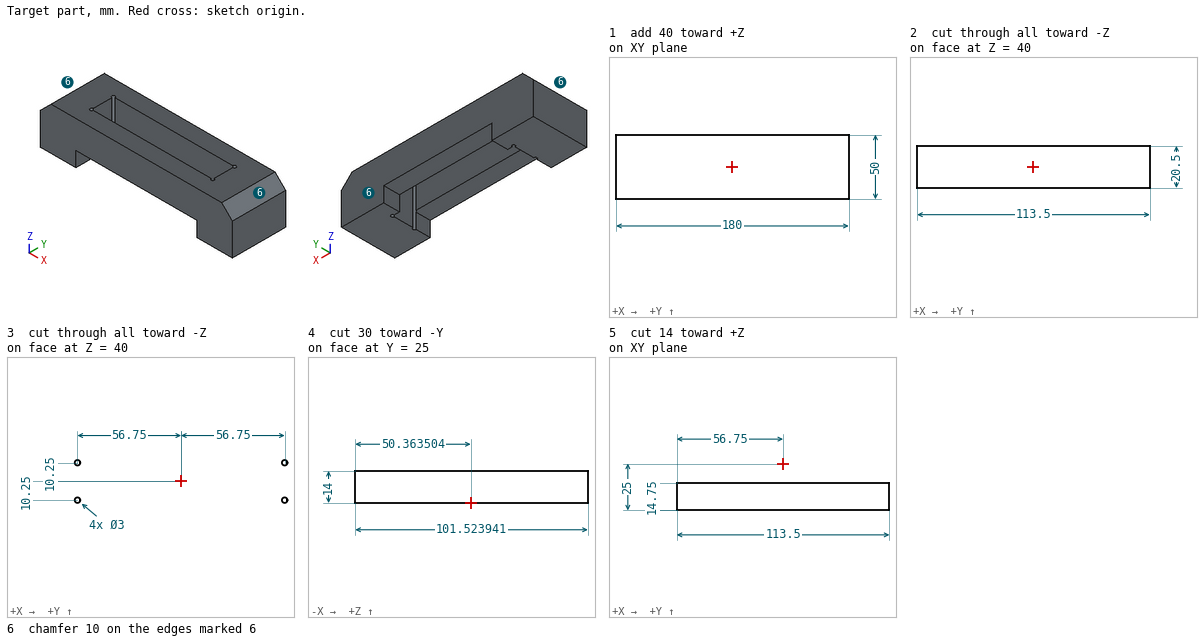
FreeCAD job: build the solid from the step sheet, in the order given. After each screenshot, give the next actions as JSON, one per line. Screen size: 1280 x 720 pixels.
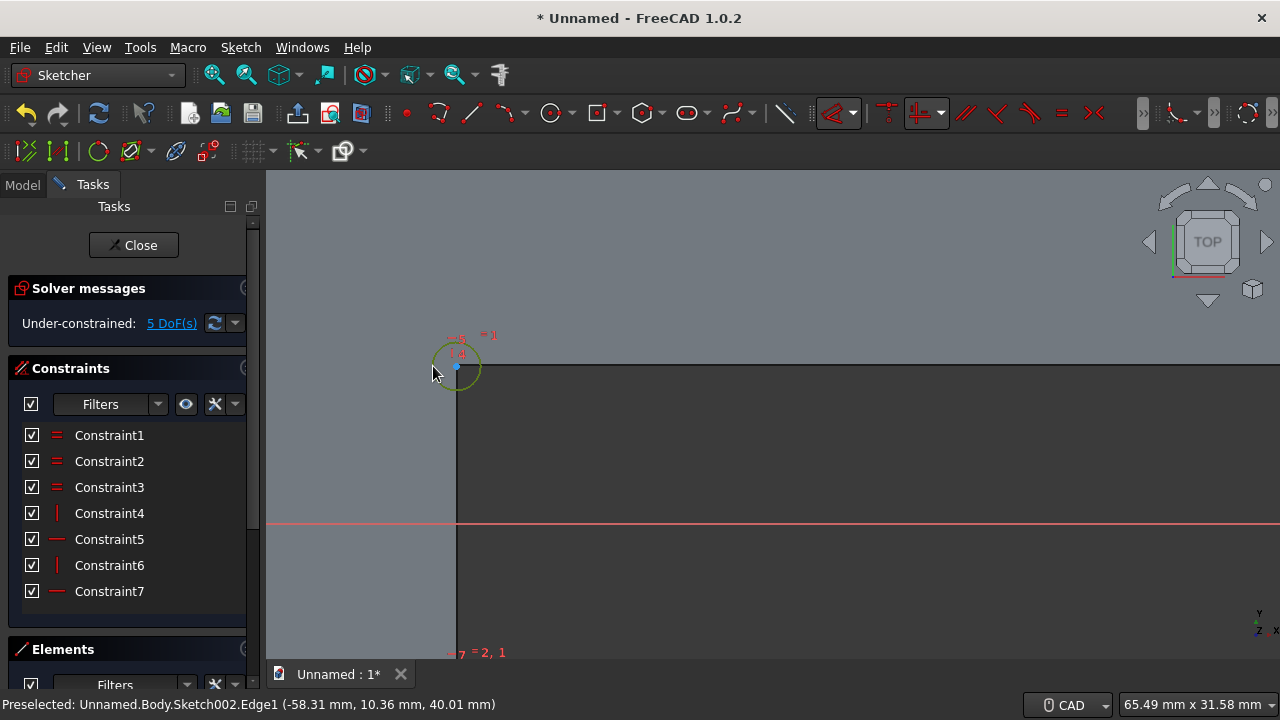
{"action": "left_click", "coordinate": [856, 114]}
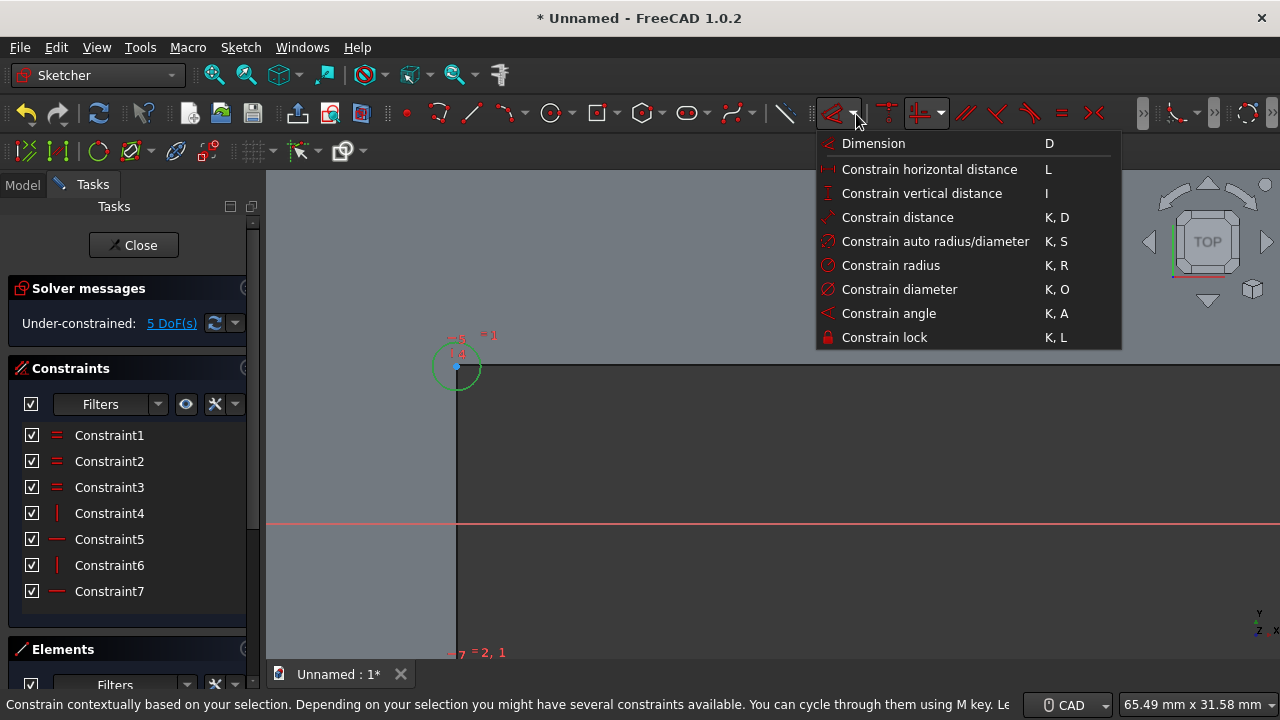
{"action": "left_click", "coordinate": [969, 289]}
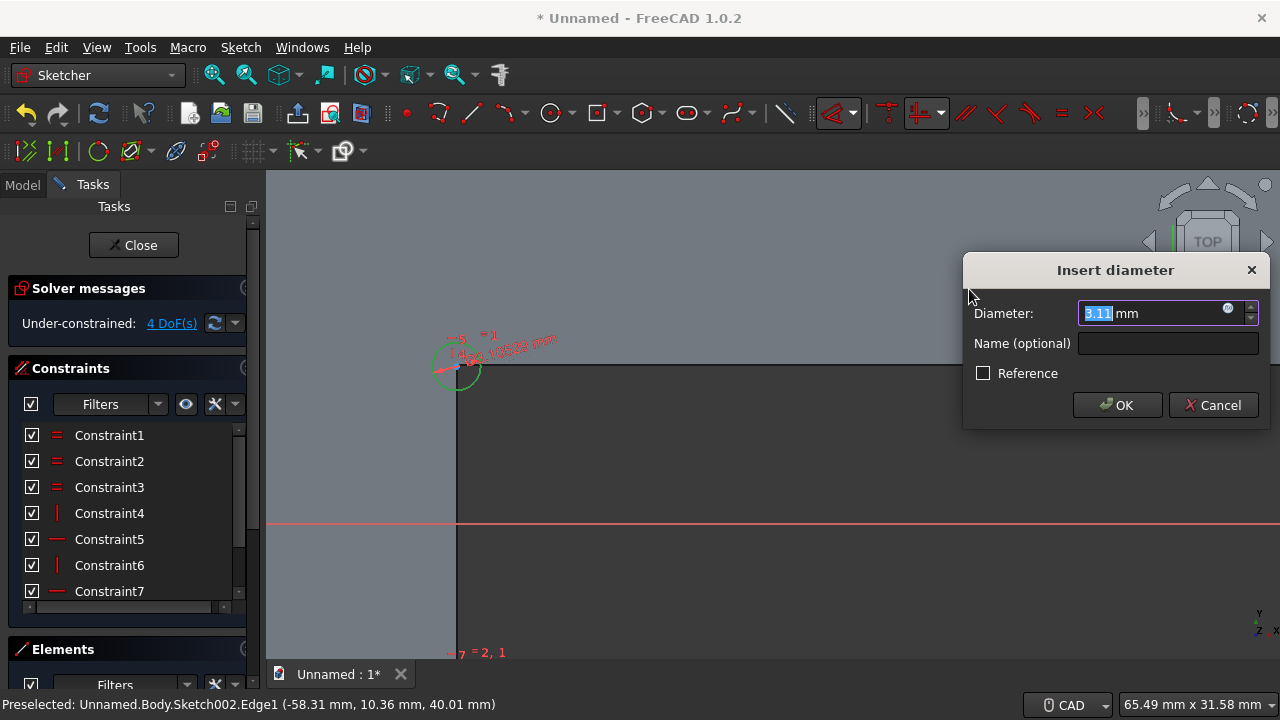
{"action": "type", "text": "3"}
{"action": "key", "text": "Return"}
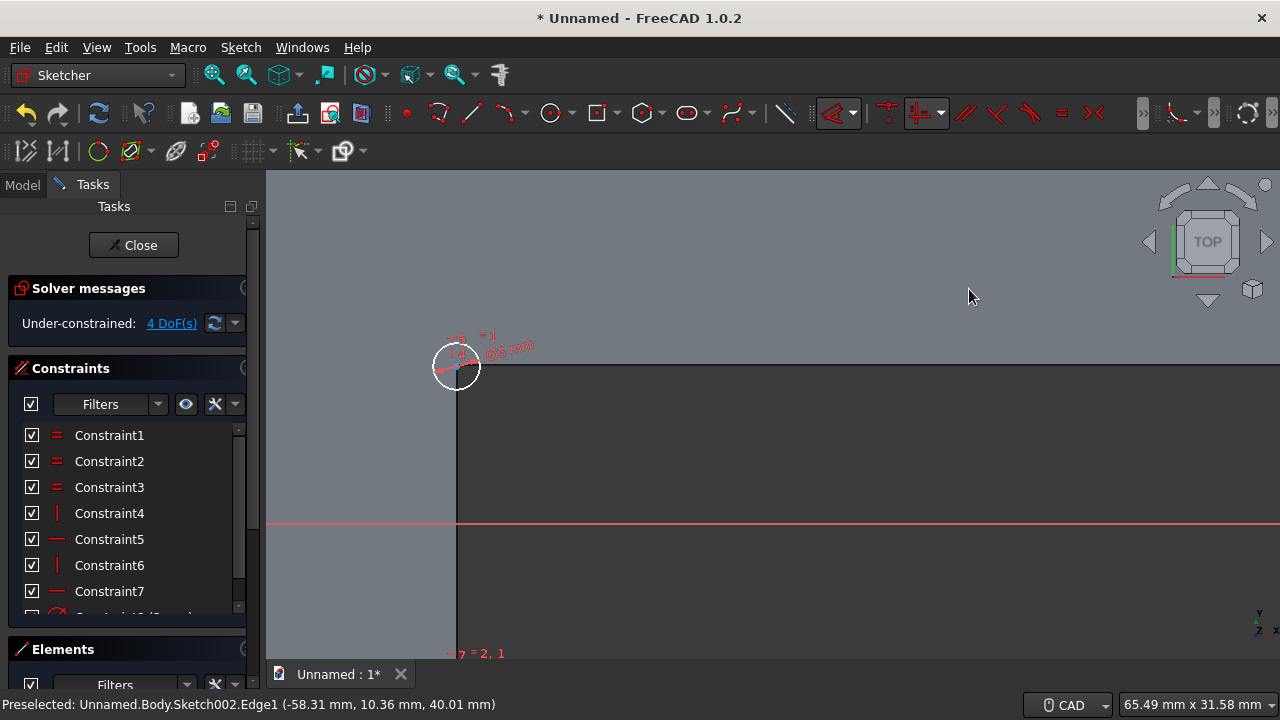
{"action": "left_click", "coordinate": [457, 366]}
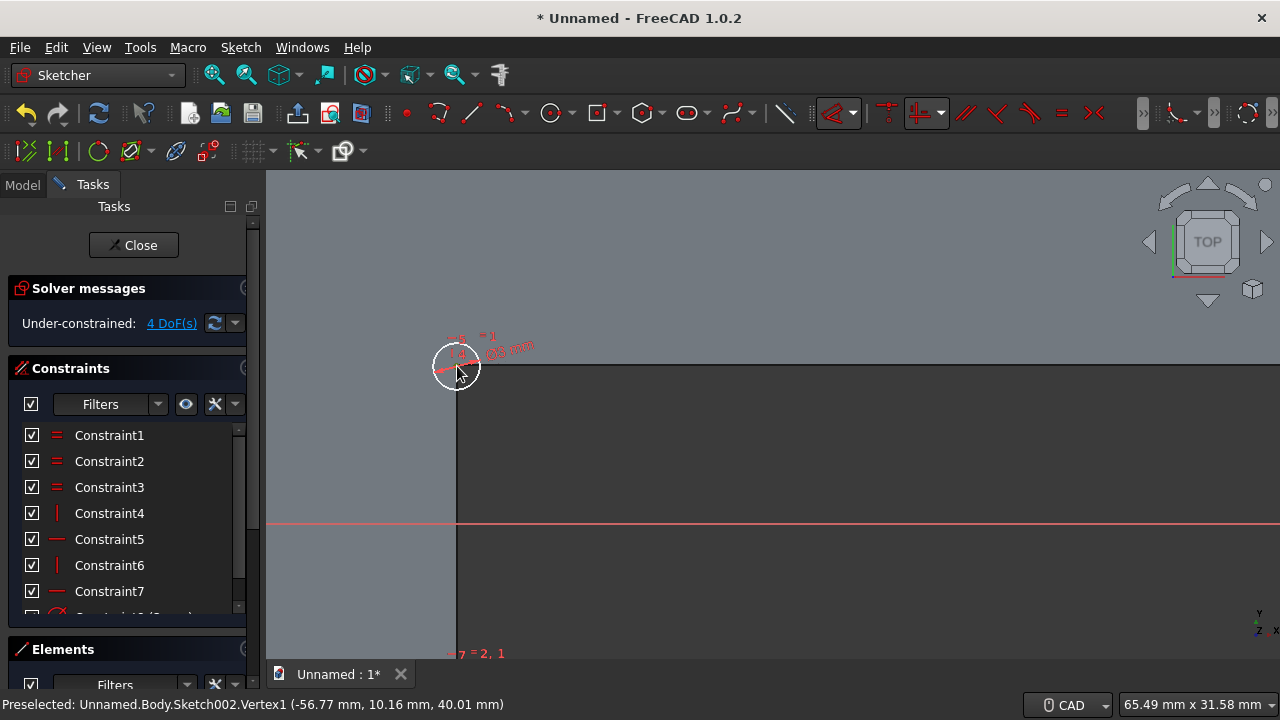
{"action": "left_click", "coordinate": [856, 114]}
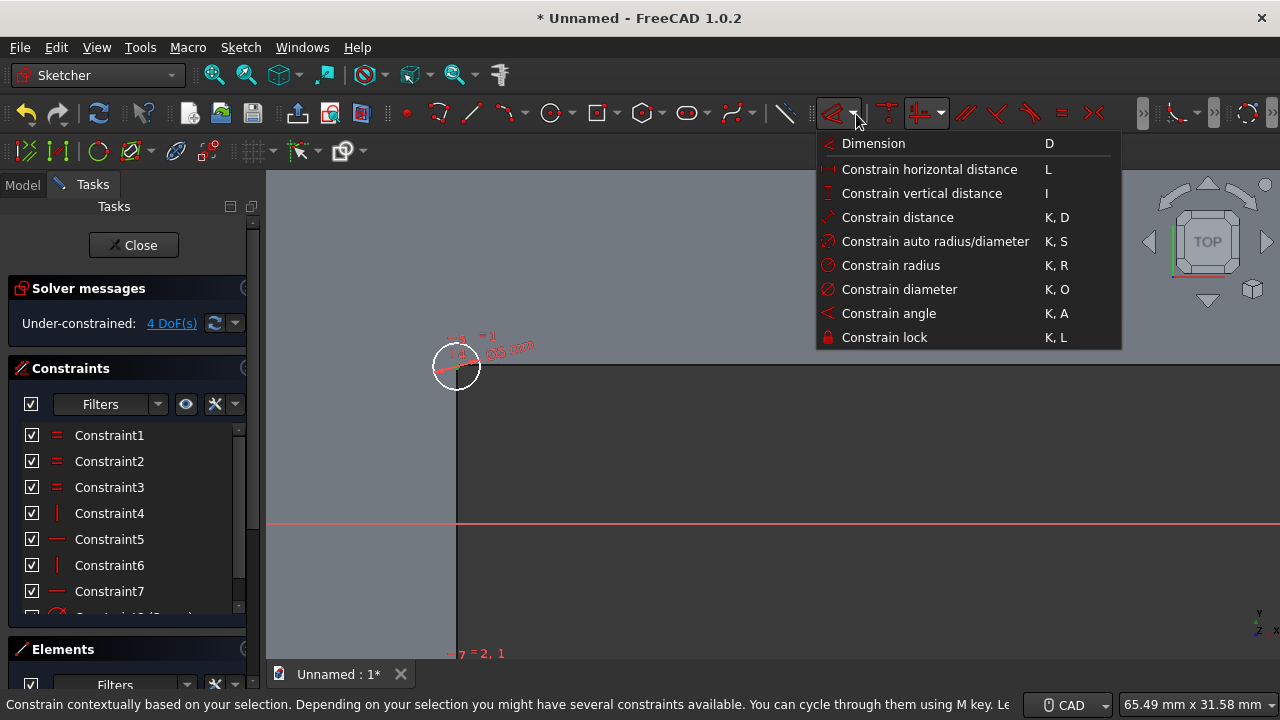
{"action": "left_click", "coordinate": [969, 169]}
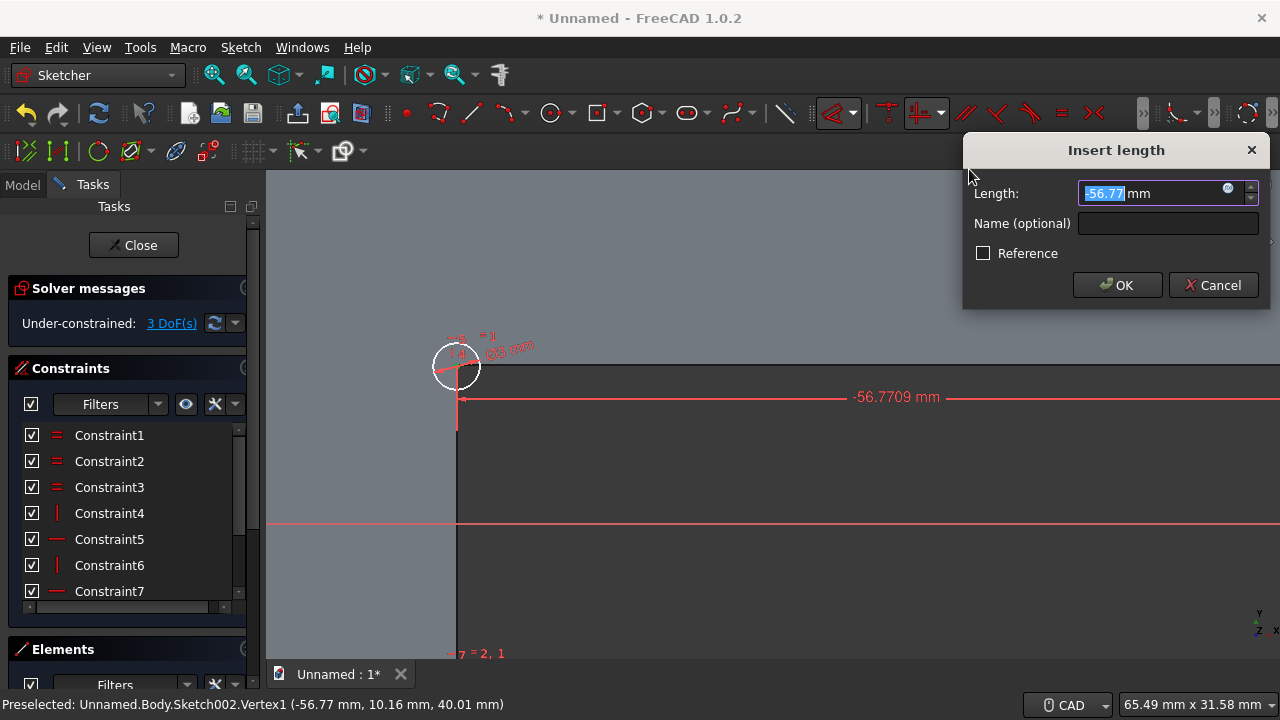
{"action": "type", "text": "-56.75"}
{"action": "key", "text": "Return"}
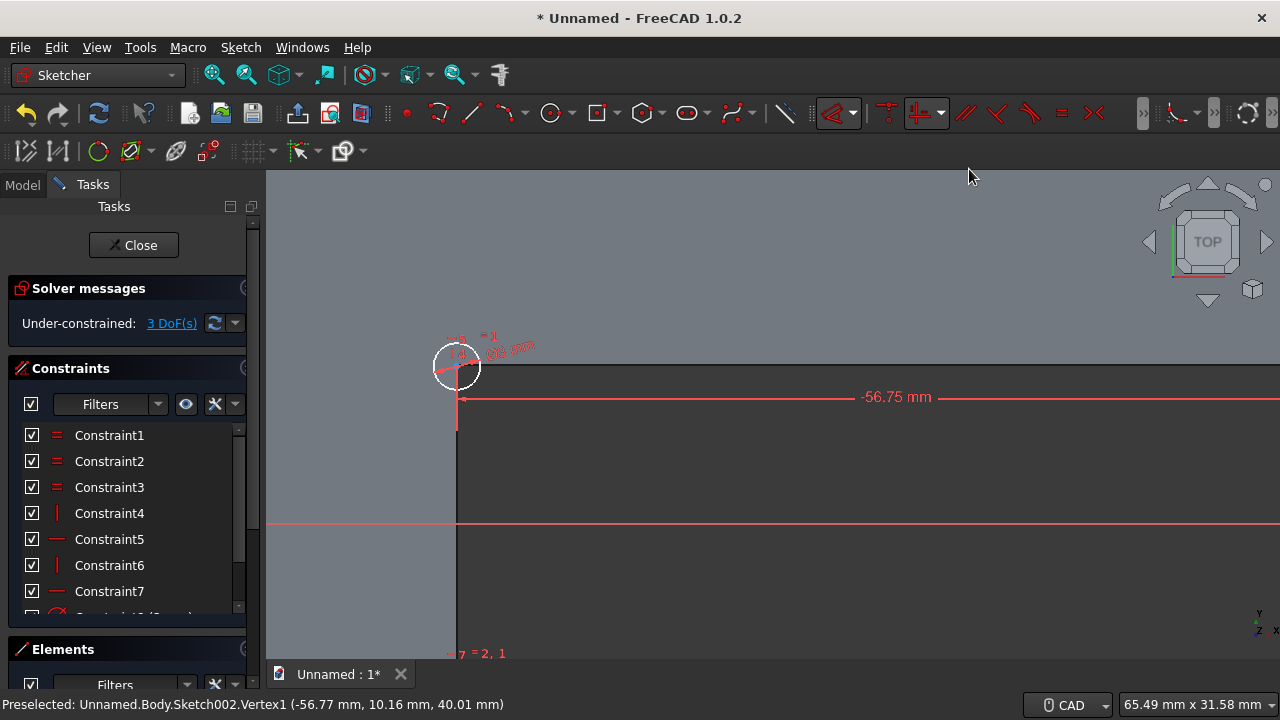
{"action": "left_click", "coordinate": [457, 366]}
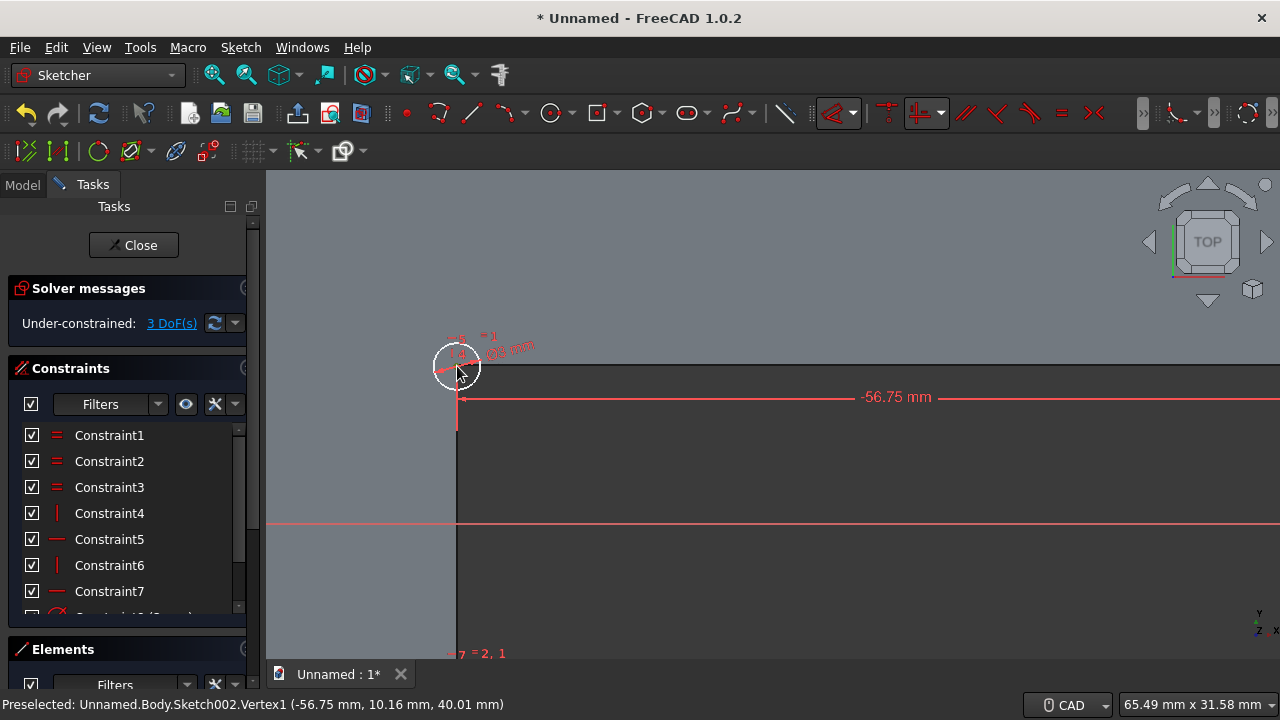
{"action": "left_click", "coordinate": [856, 114]}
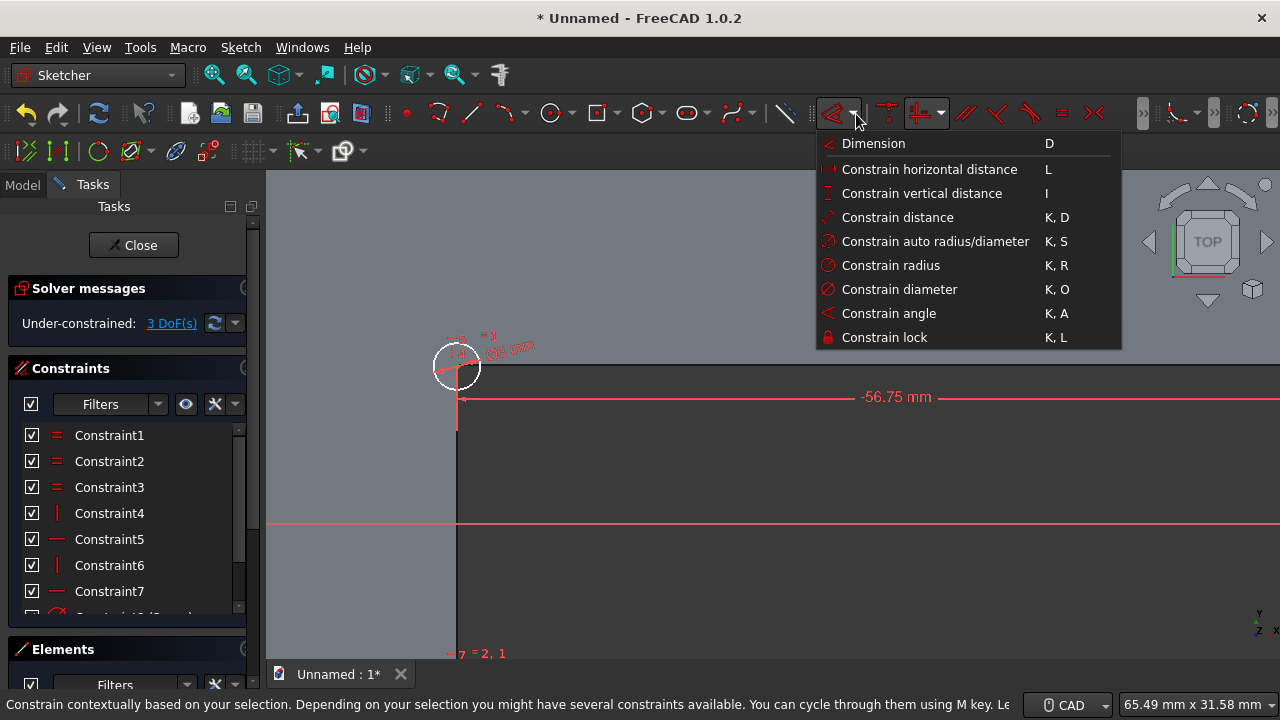
{"action": "left_click", "coordinate": [969, 193]}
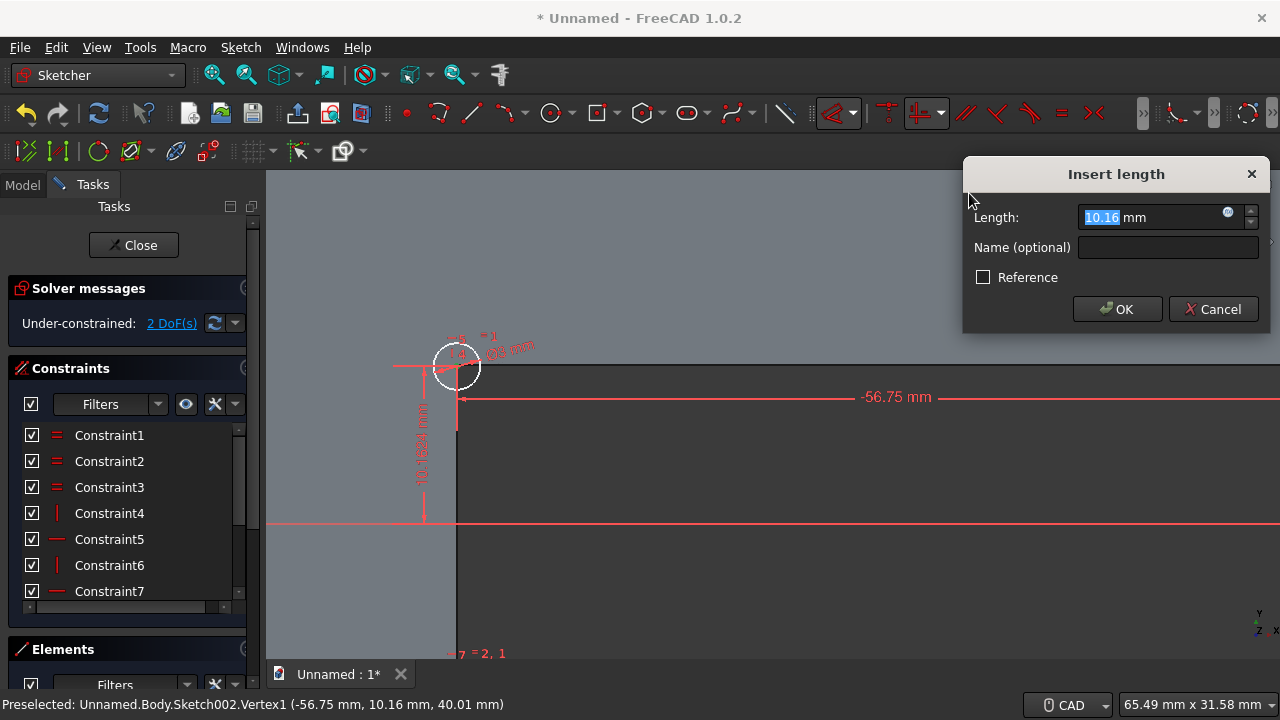
{"action": "type", "text": "10.25"}
{"action": "key", "text": "Return"}